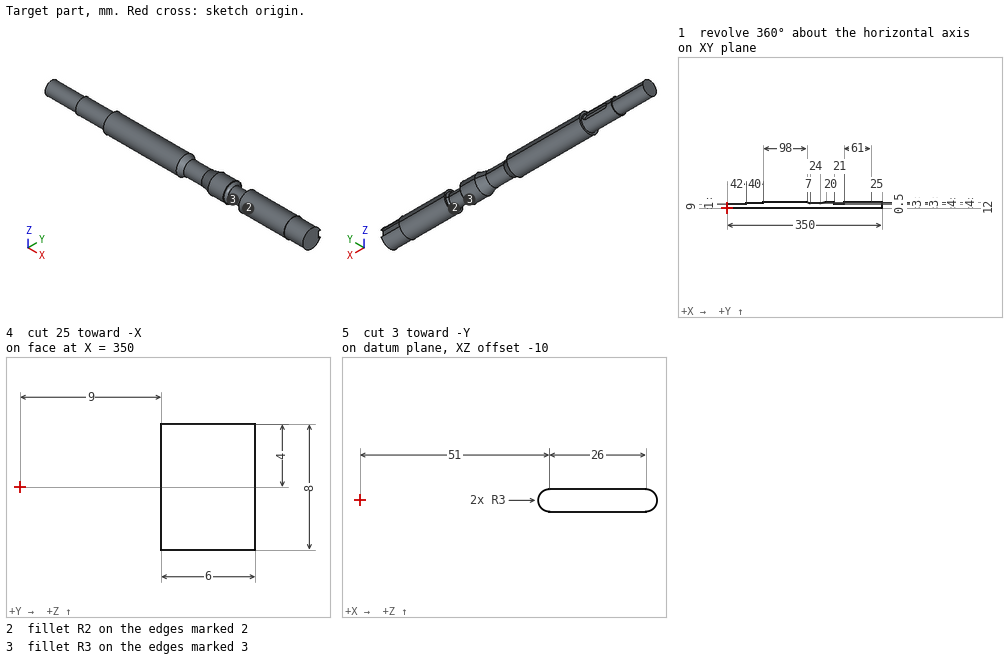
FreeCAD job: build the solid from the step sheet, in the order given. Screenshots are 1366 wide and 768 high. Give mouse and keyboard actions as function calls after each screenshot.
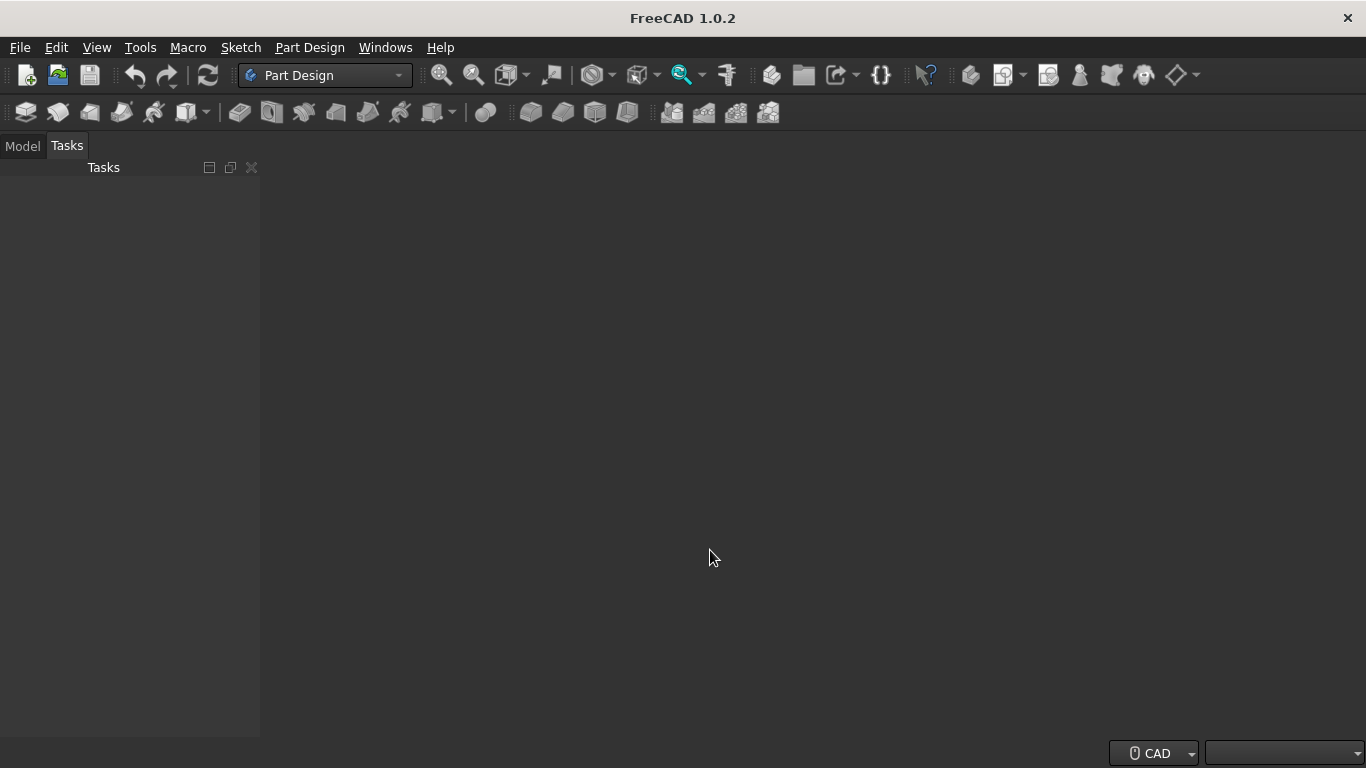
click(26, 76)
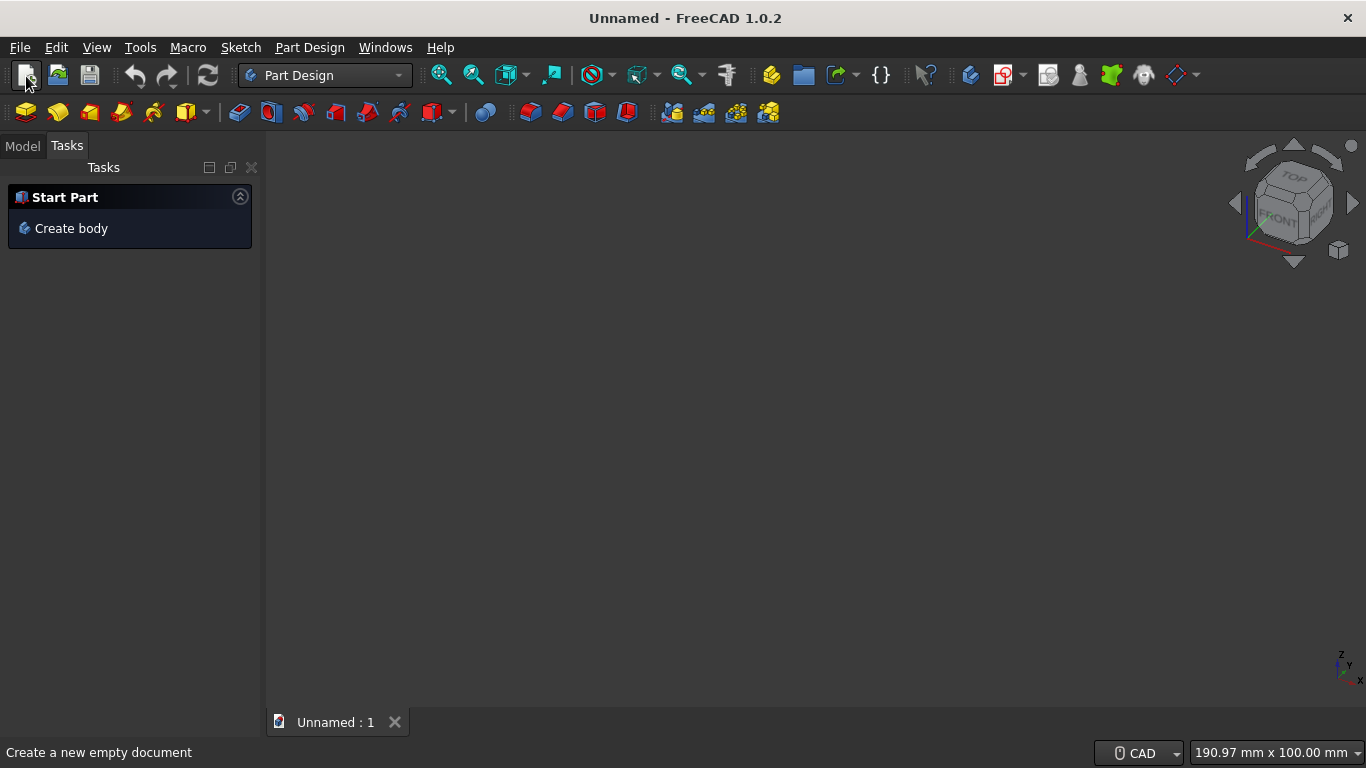
click(1004, 76)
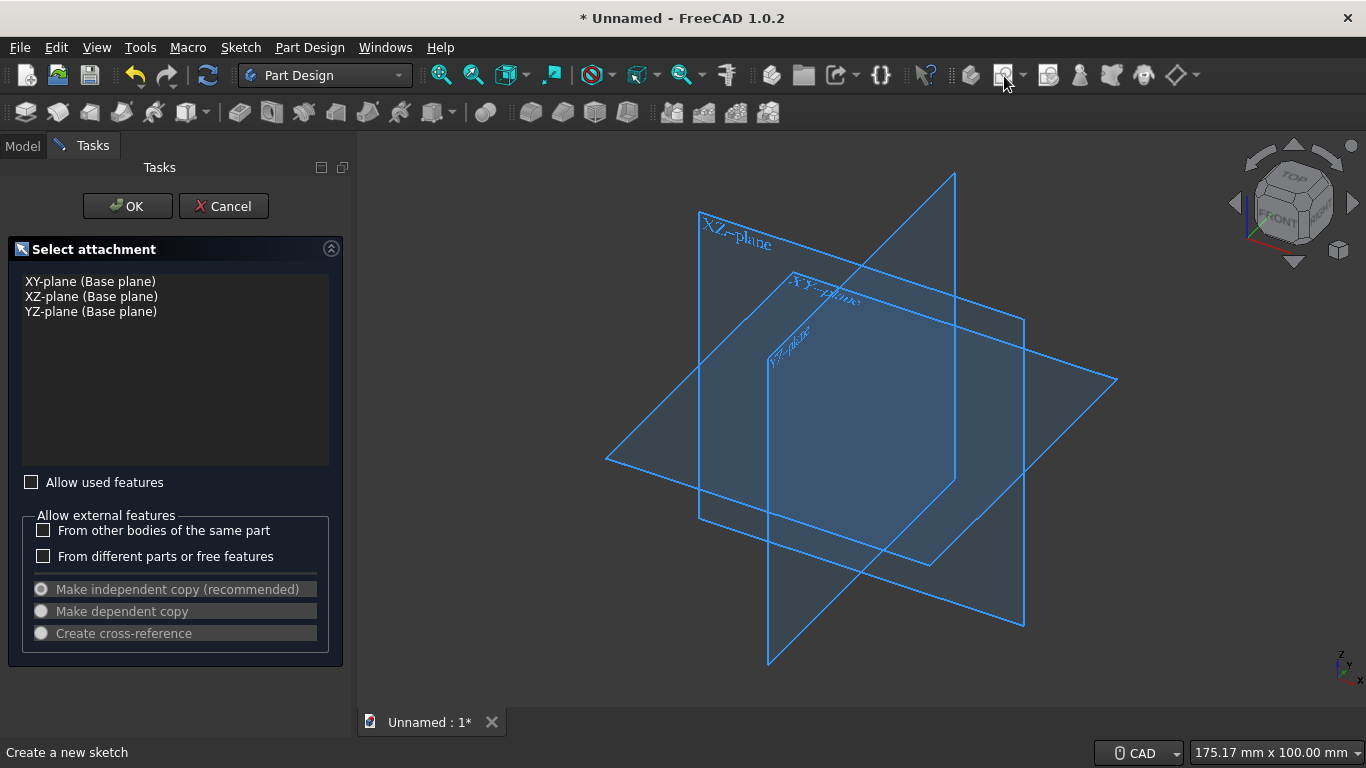
click(82, 282)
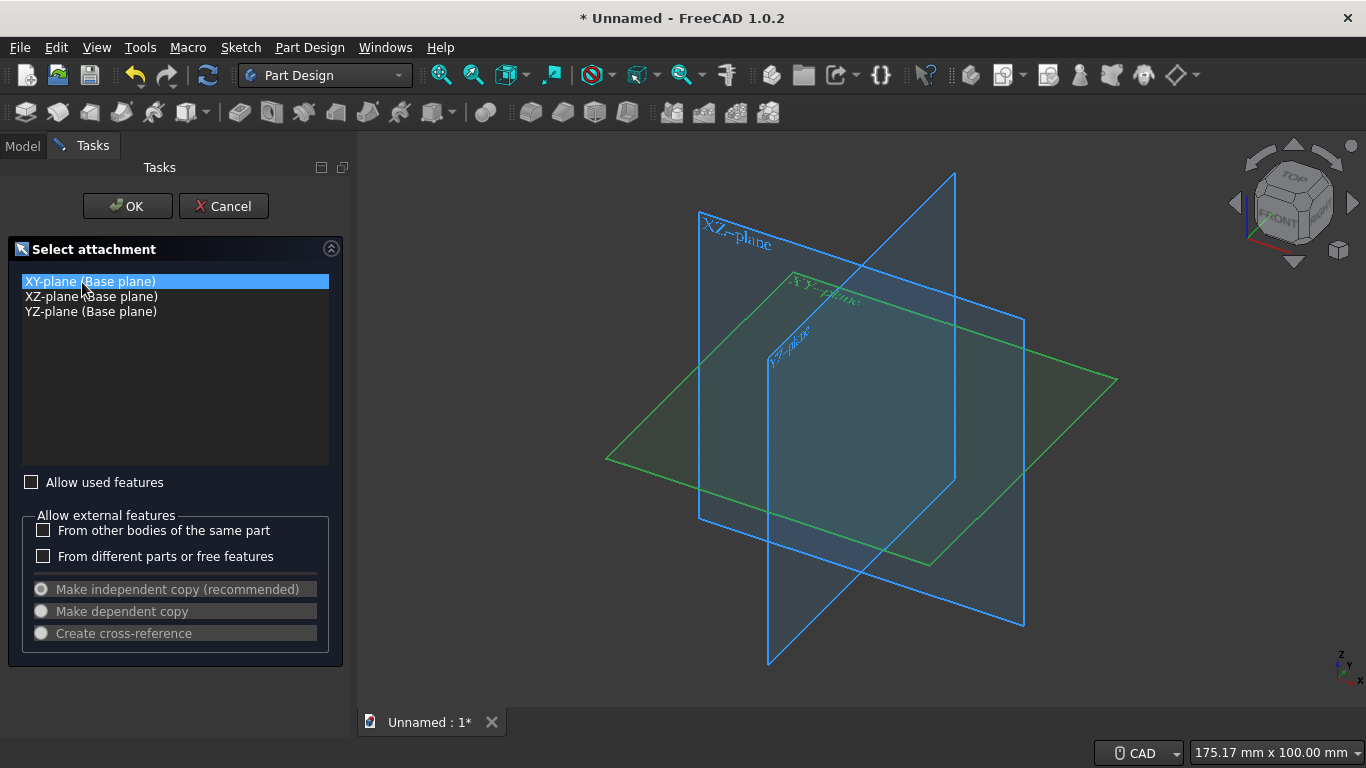
click(128, 206)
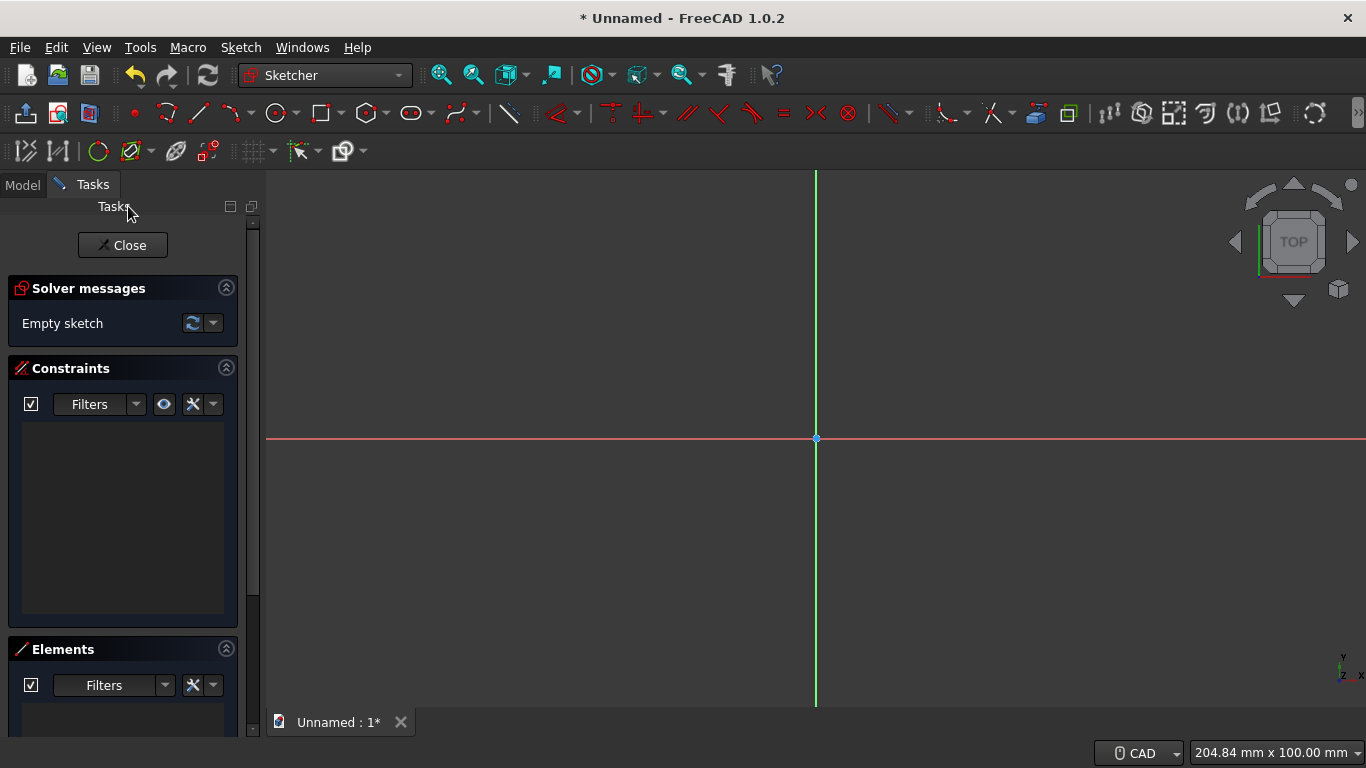
scroll(313, 453, down, 6)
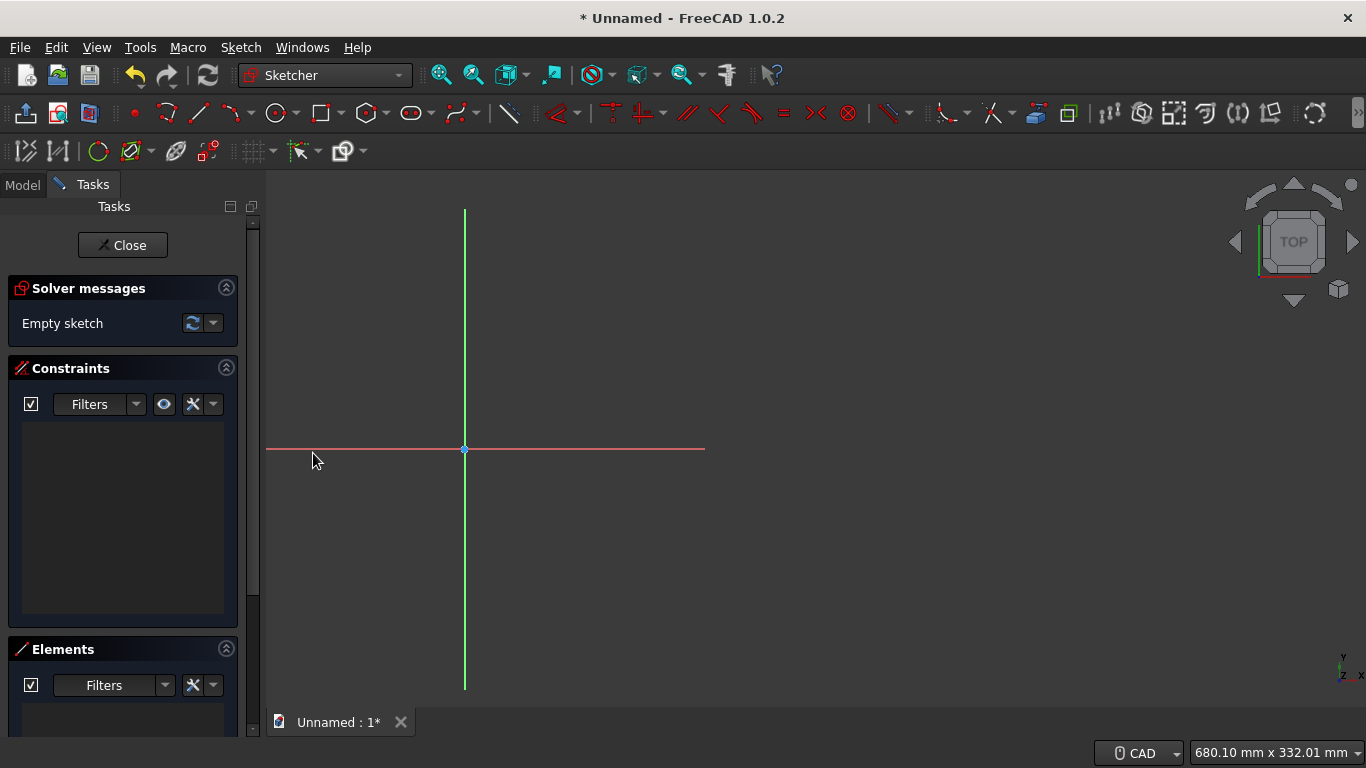
click(168, 114)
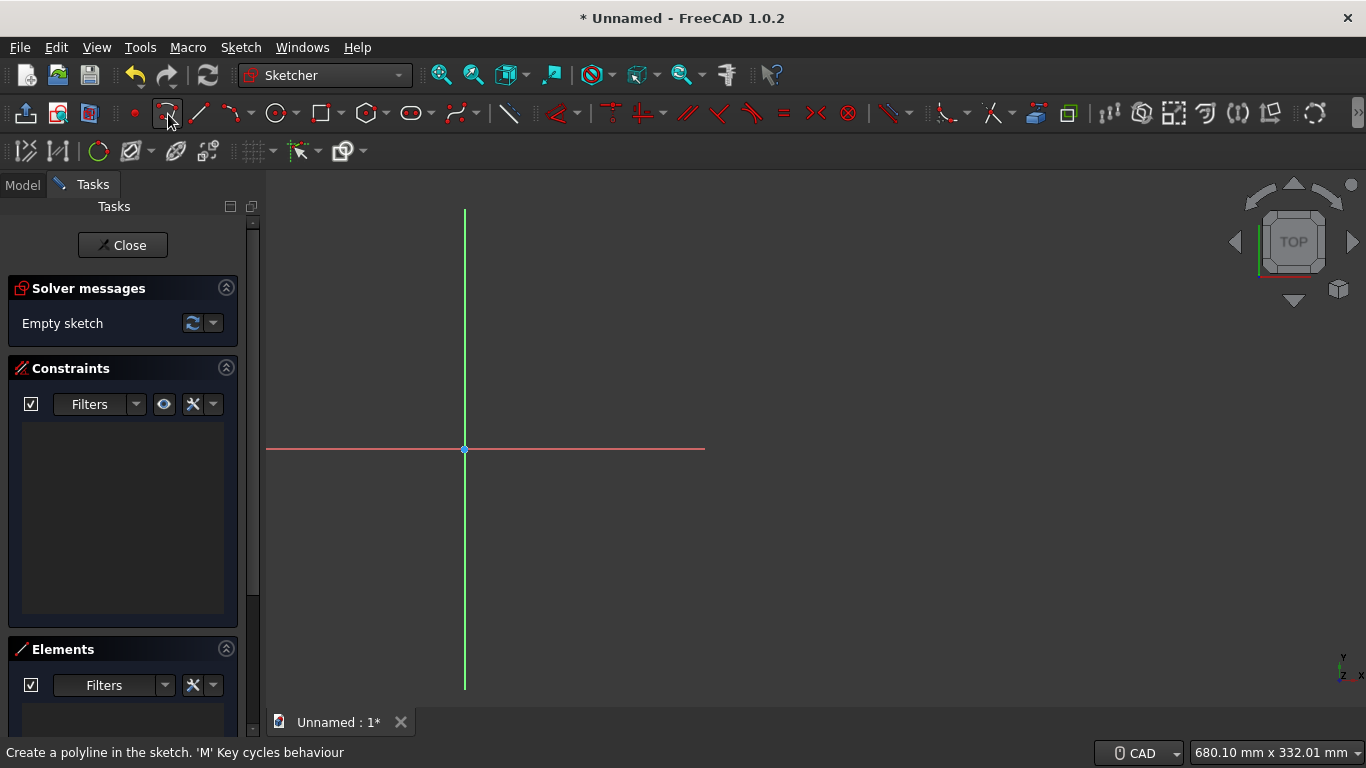
click(465, 449)
click(1031, 440)
click(1031, 430)
click(990, 430)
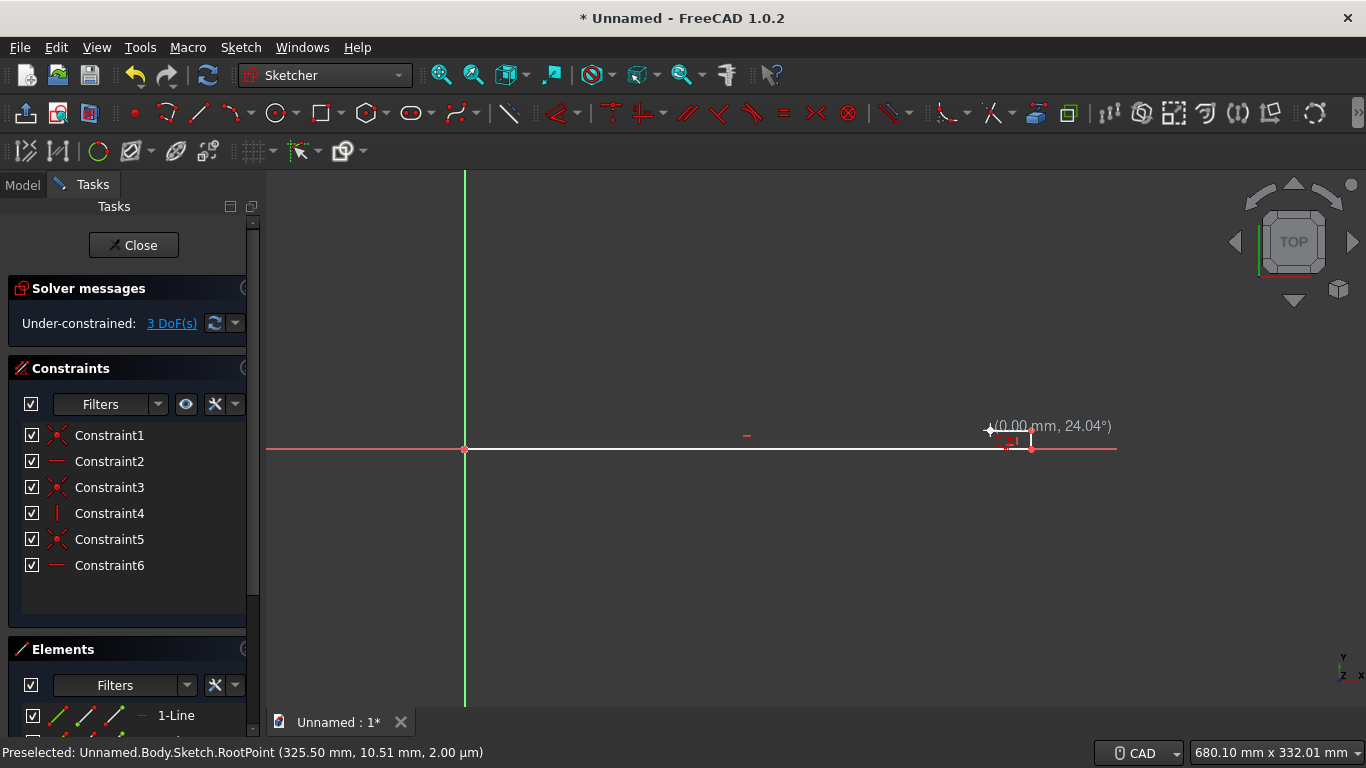
scroll(990, 429, up, 15)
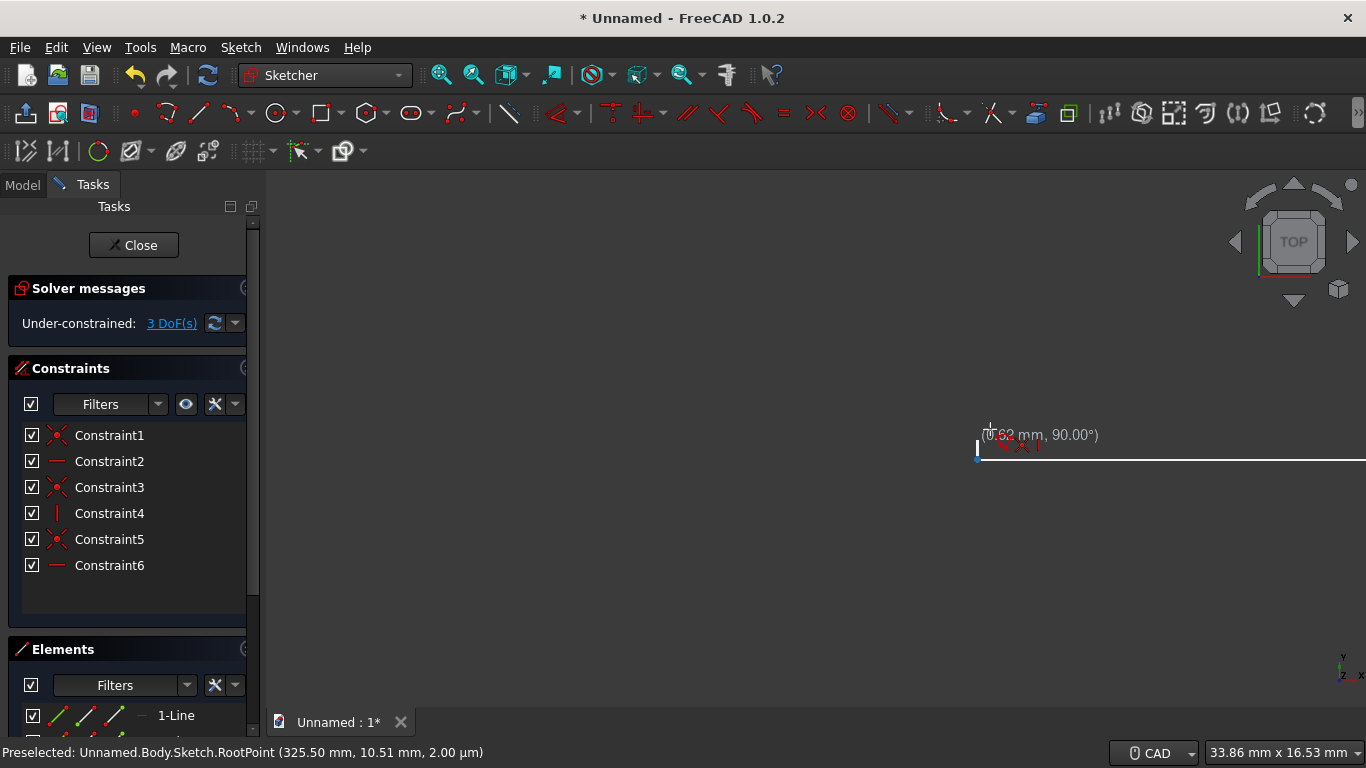
click(977, 415)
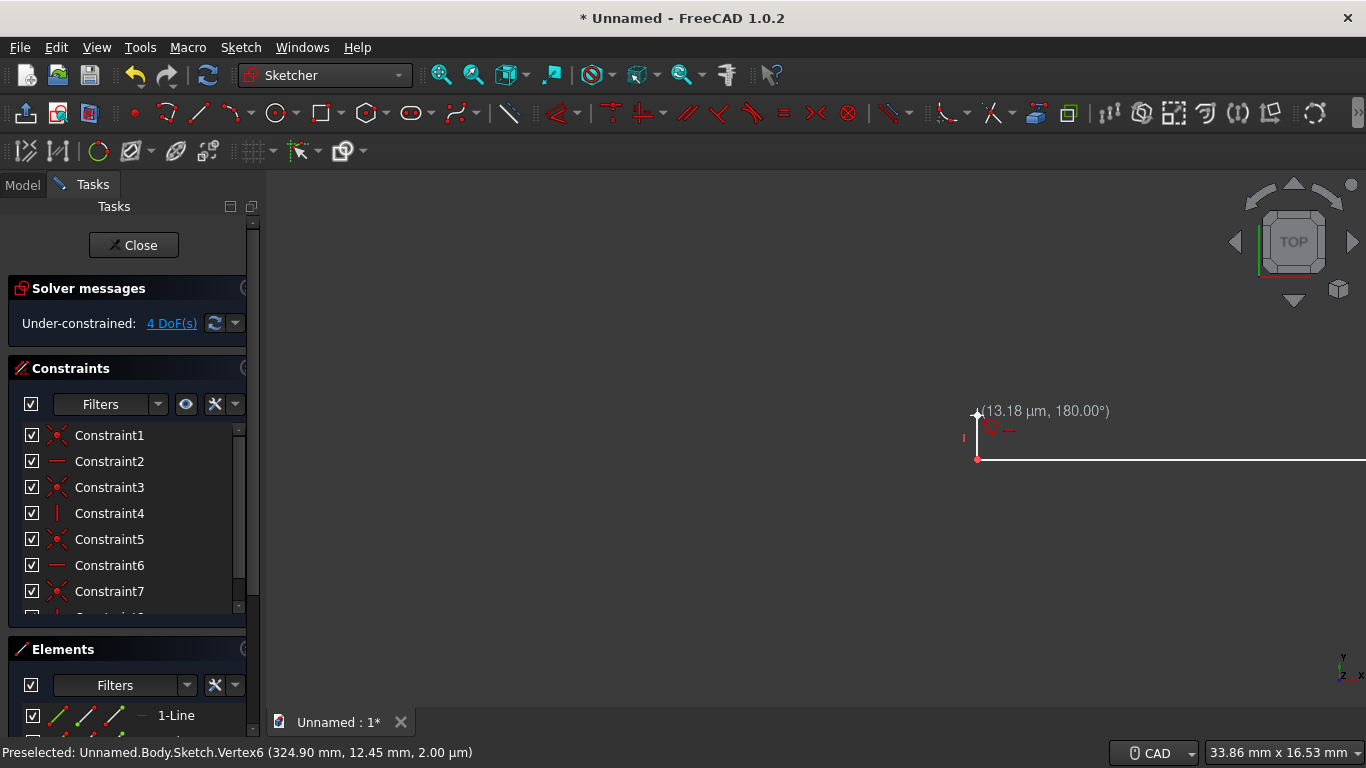
scroll(1048, 427, down, 14)